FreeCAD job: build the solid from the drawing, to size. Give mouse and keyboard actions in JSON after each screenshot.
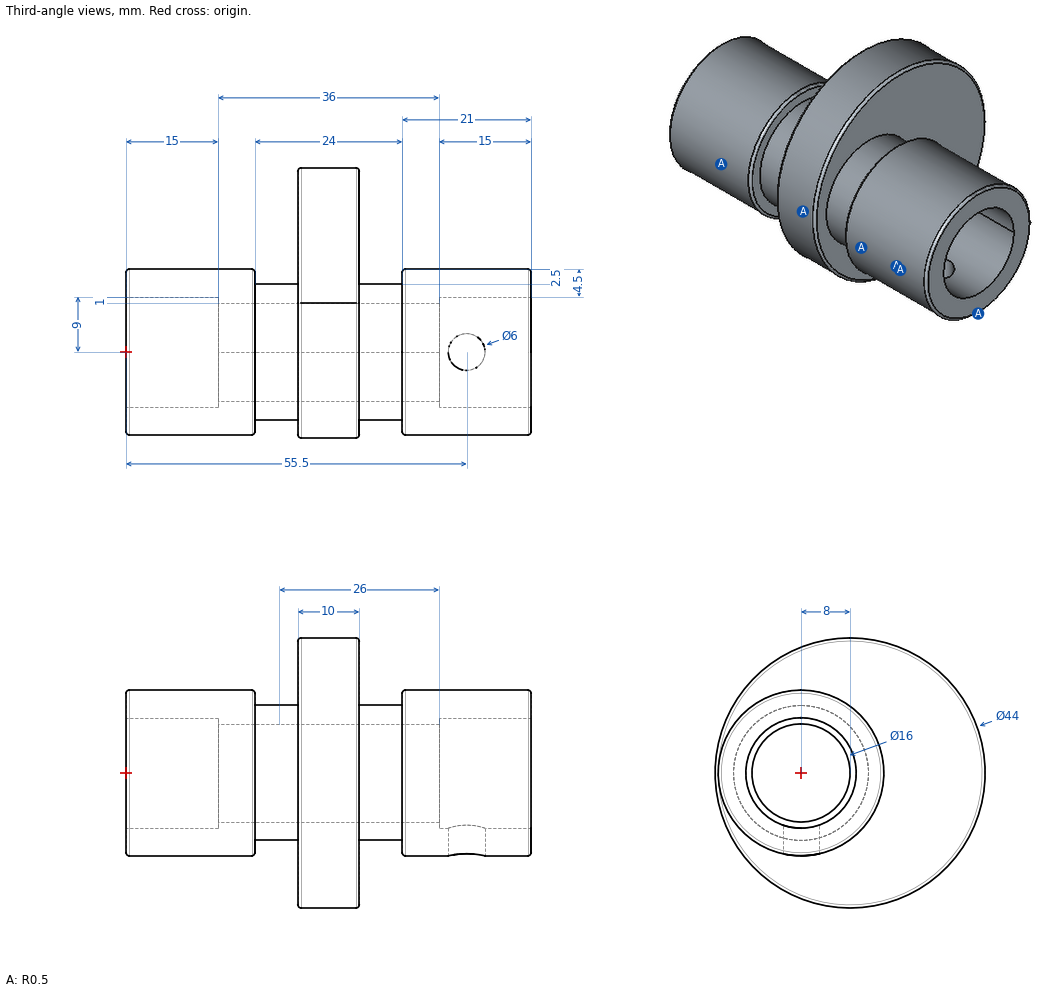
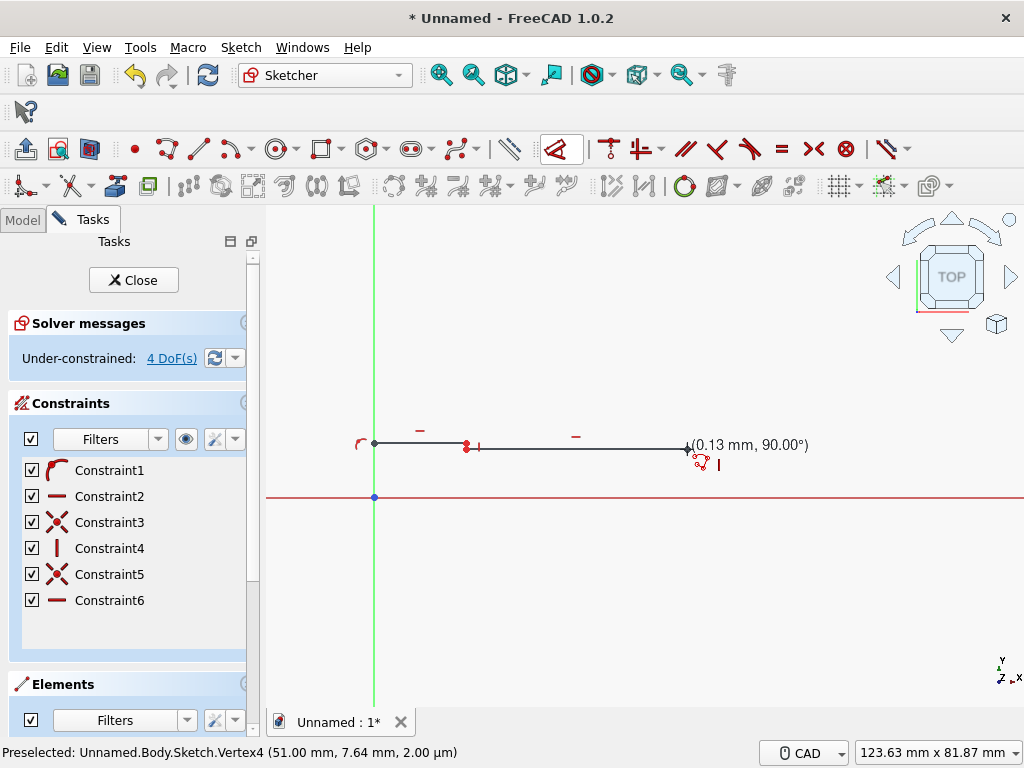
{"action": "scroll", "coordinate": [687, 443], "scroll_direction": "up", "scroll_amount": 5}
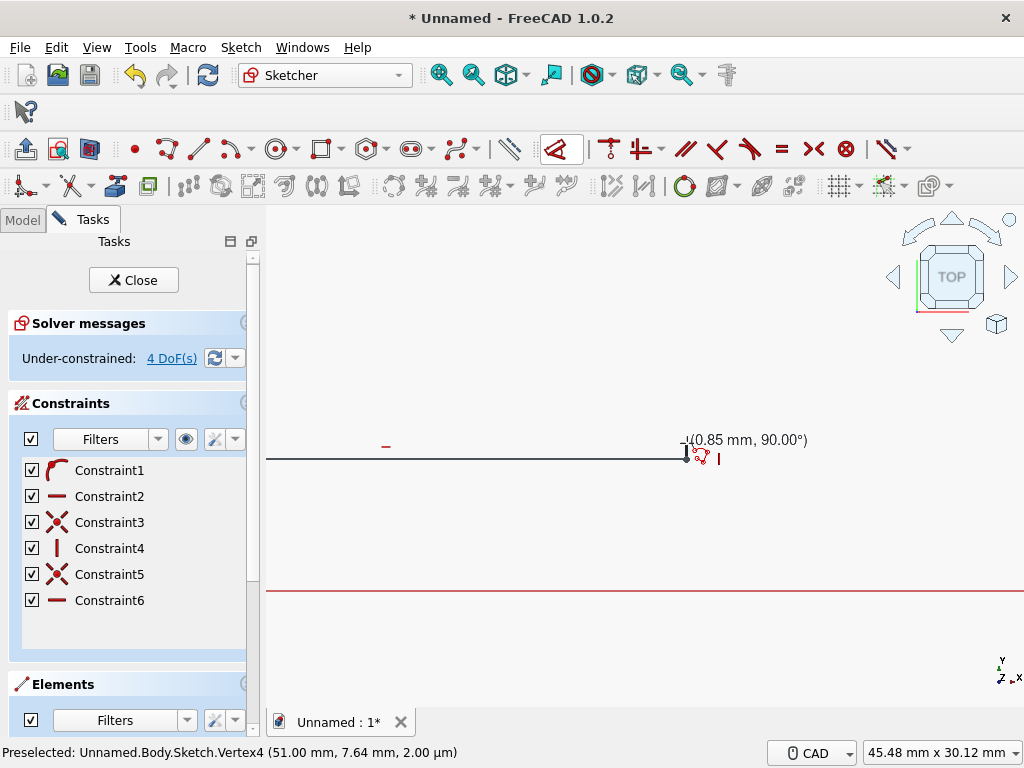
{"action": "left_click", "coordinate": [686, 441]}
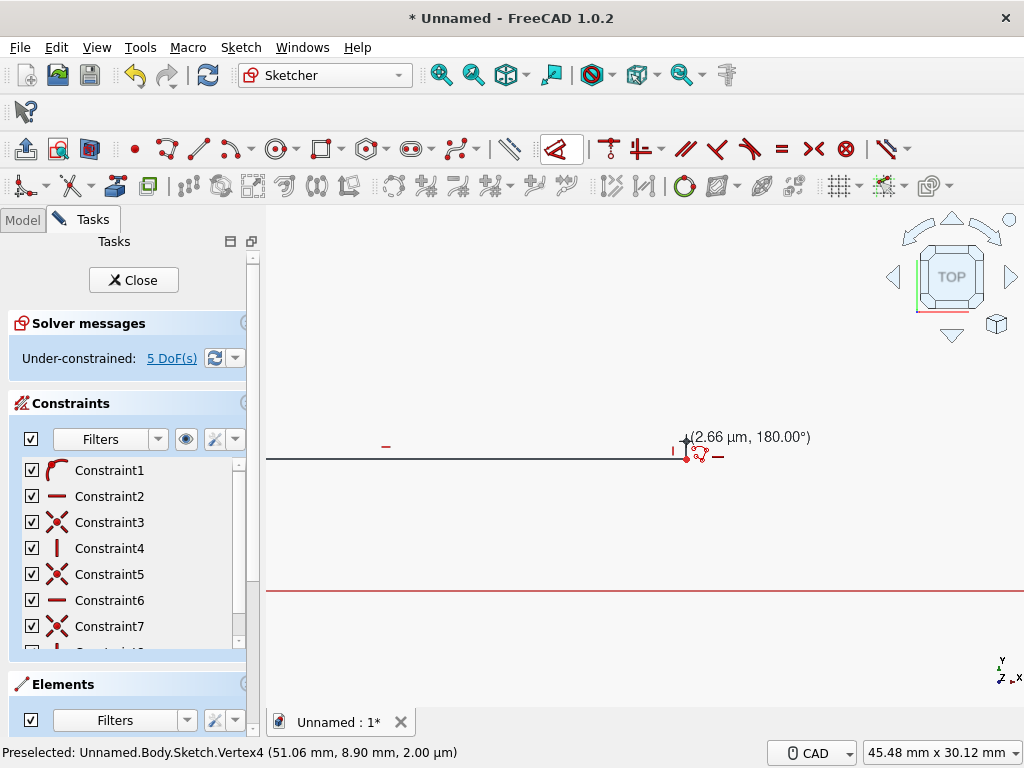
{"action": "scroll", "coordinate": [687, 443], "scroll_direction": "down", "scroll_amount": 5}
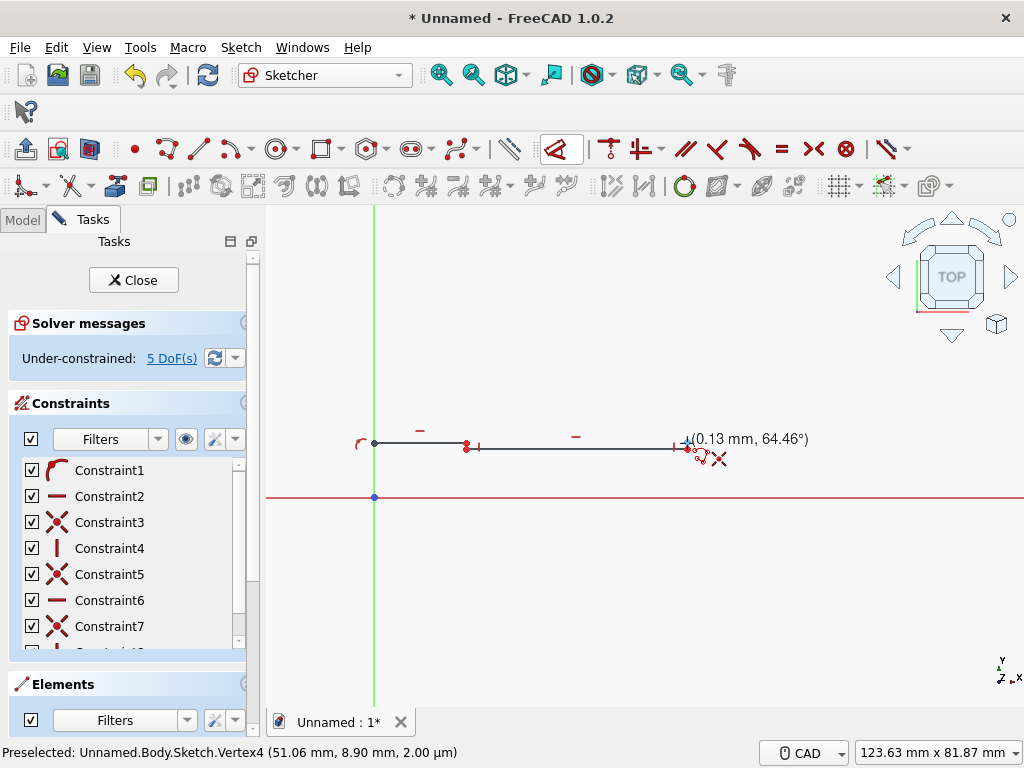
{"action": "left_click", "coordinate": [779, 443]}
{"action": "left_click", "coordinate": [779, 415]}
{"action": "left_click", "coordinate": [650, 415]}
{"action": "left_click", "coordinate": [650, 430]}
{"action": "left_click", "coordinate": [503, 430]}
{"action": "left_click", "coordinate": [503, 415]}
{"action": "left_click", "coordinate": [383, 415]}
{"action": "left_click", "coordinate": [374, 443]}
{"action": "key", "text": "Escape"}
{"action": "key", "text": "Escape"}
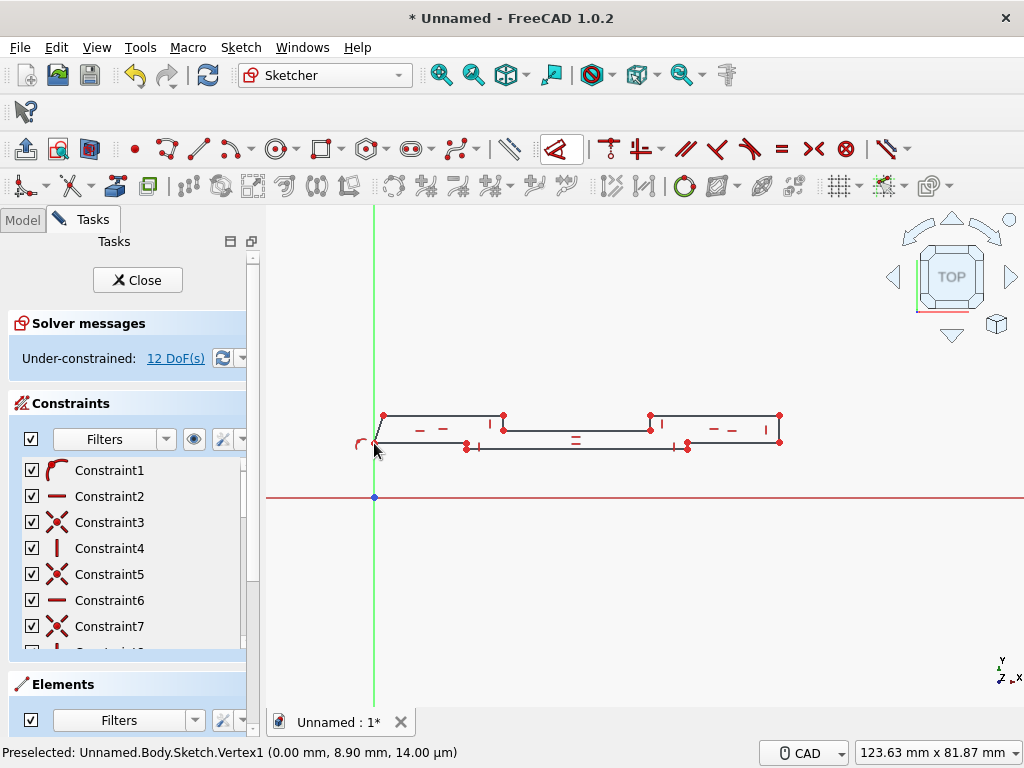
{"action": "scroll", "coordinate": [378, 432], "scroll_direction": "up", "scroll_amount": 2}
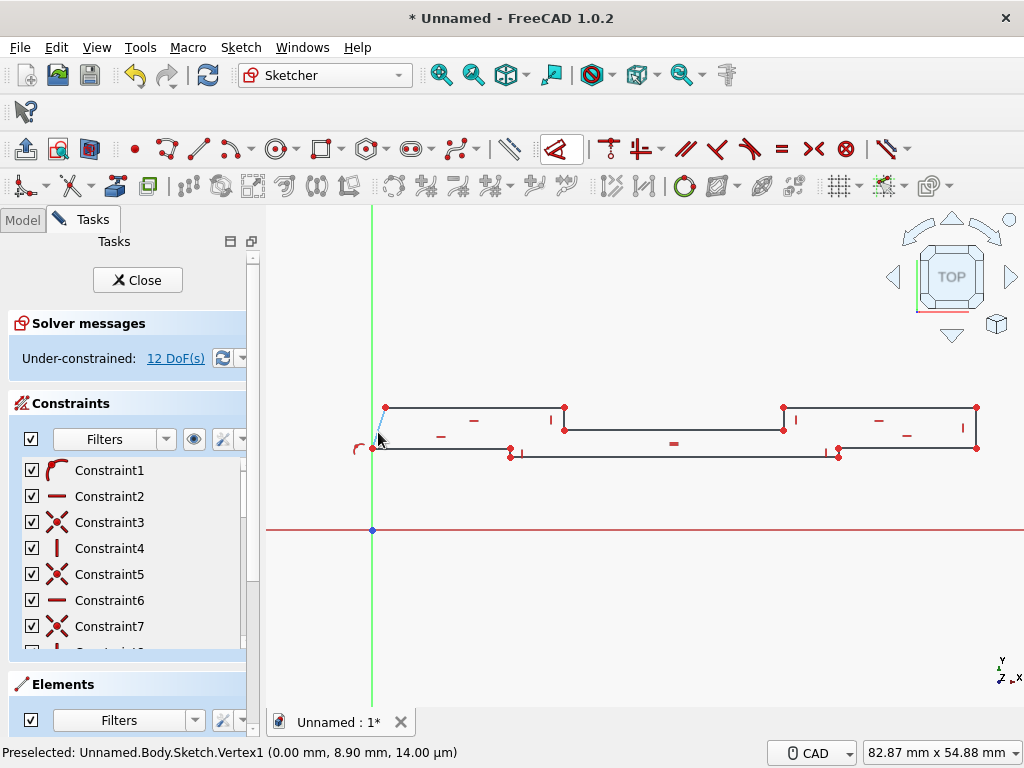
{"action": "left_click", "coordinate": [378, 432]}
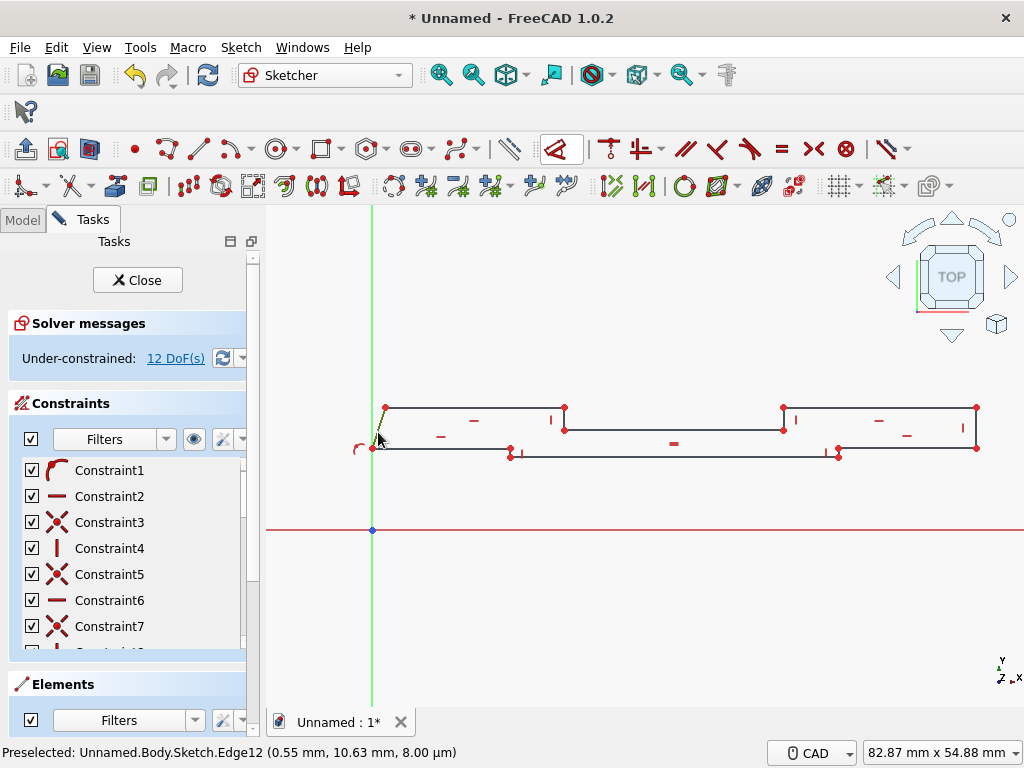
{"action": "key", "text": "v"}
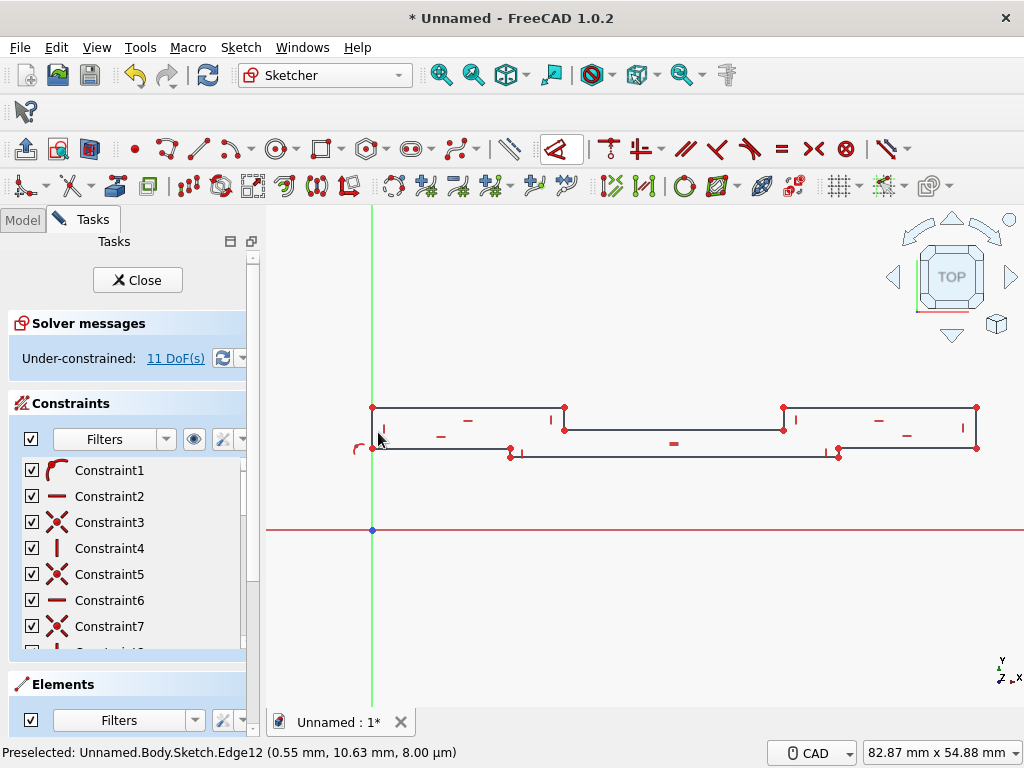
{"action": "left_click", "coordinate": [556, 150]}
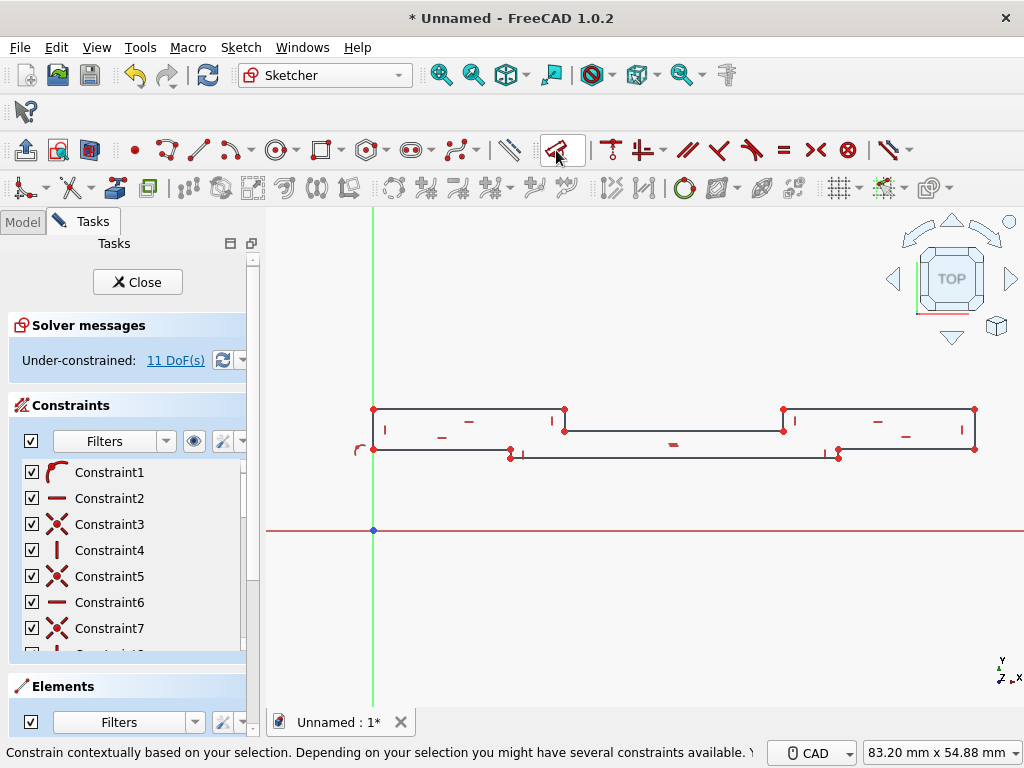
{"action": "scroll", "coordinate": [511, 454], "scroll_direction": "up", "scroll_amount": 8}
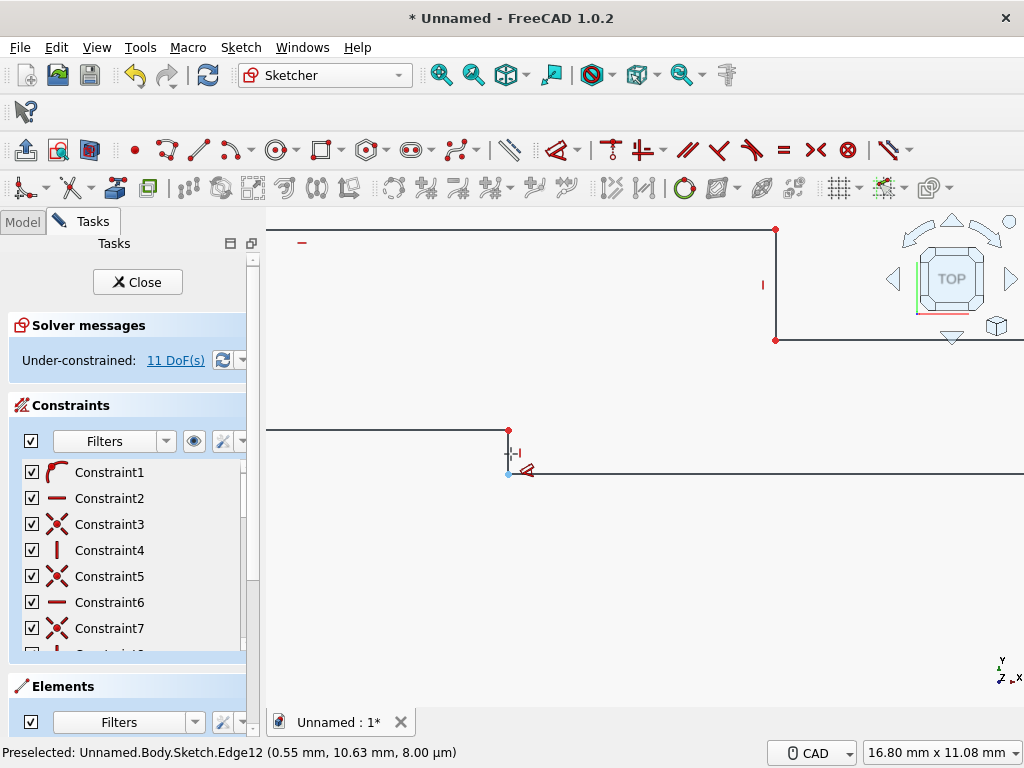
{"action": "left_click", "coordinate": [508, 452]}
{"action": "left_click", "coordinate": [474, 452]}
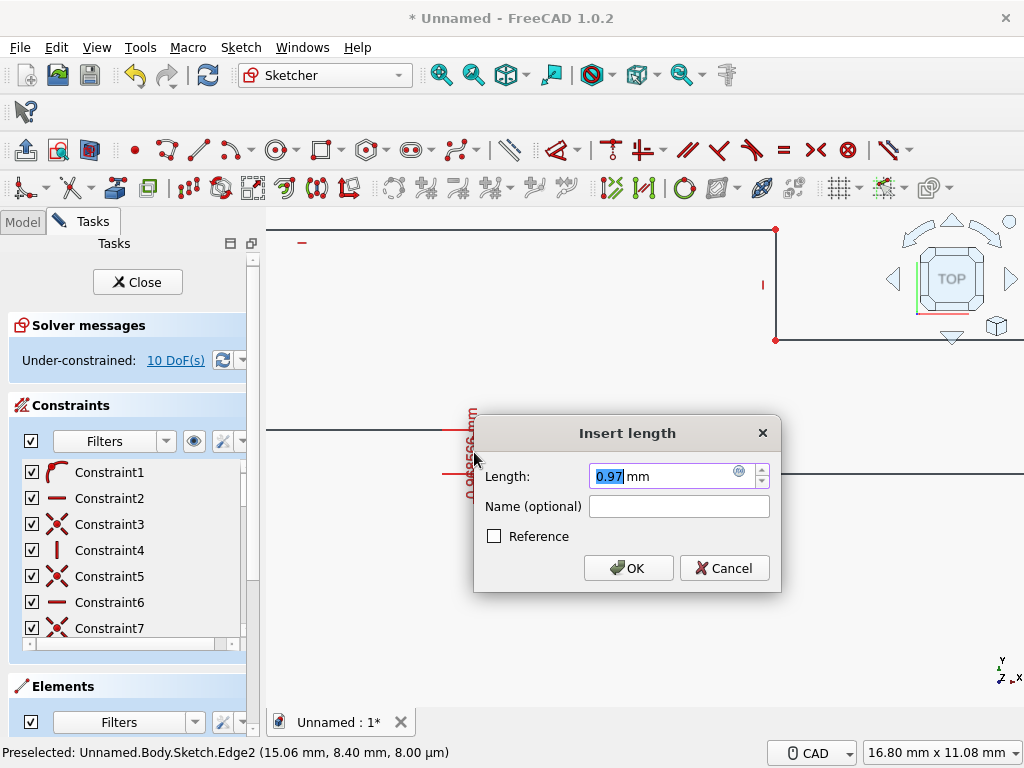
{"action": "type", "text": "1"}
{"action": "key", "text": "Return"}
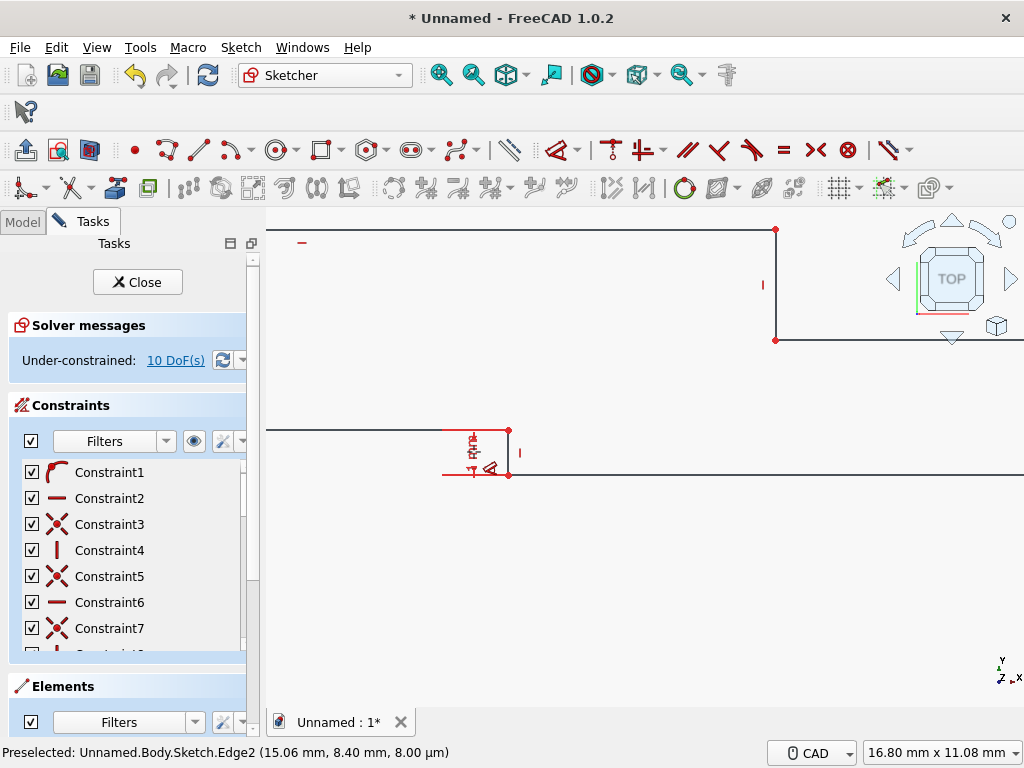
{"action": "scroll", "coordinate": [460, 446], "scroll_direction": "down", "scroll_amount": 10}